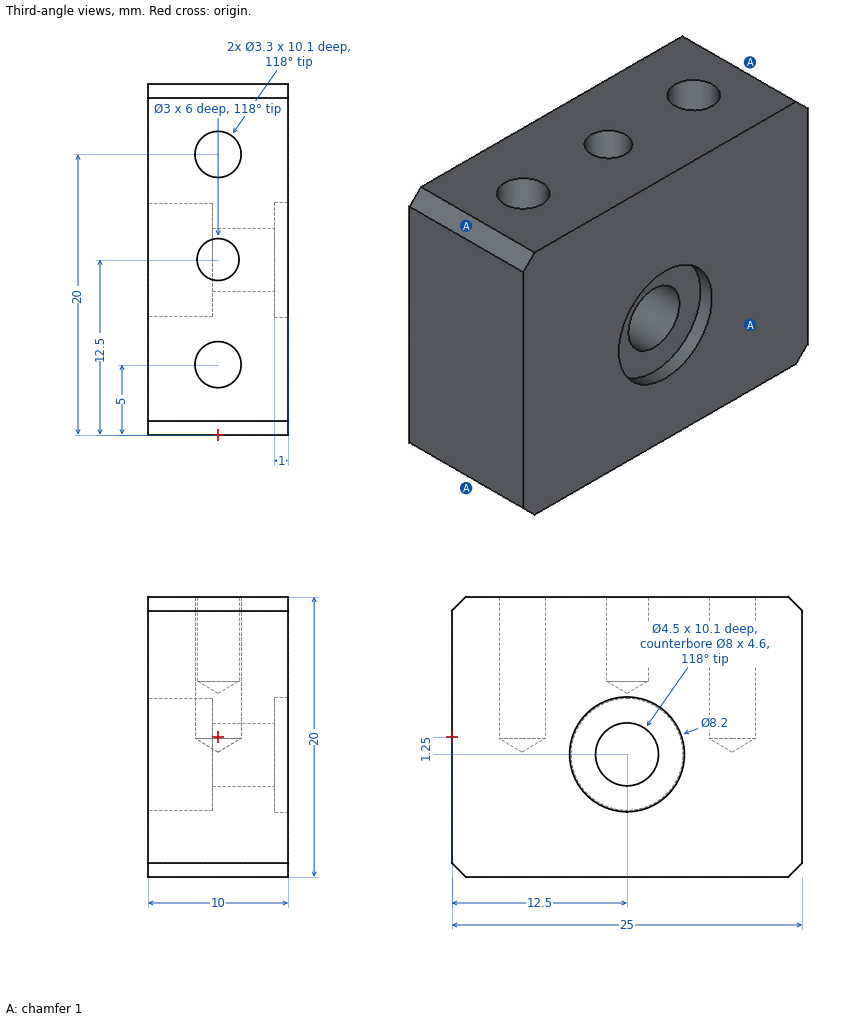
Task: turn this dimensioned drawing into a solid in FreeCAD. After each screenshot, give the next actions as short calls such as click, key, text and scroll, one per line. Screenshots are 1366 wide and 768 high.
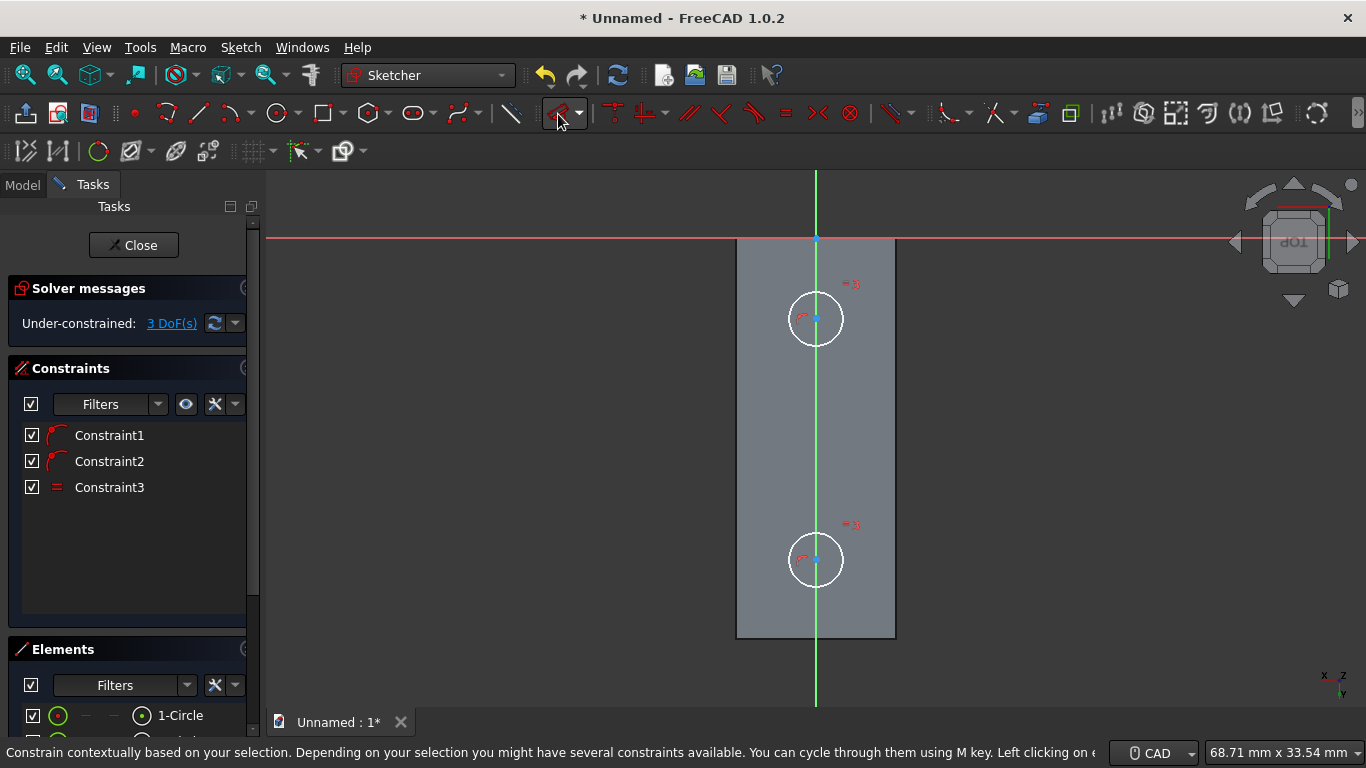
click(835, 541)
click(858, 518)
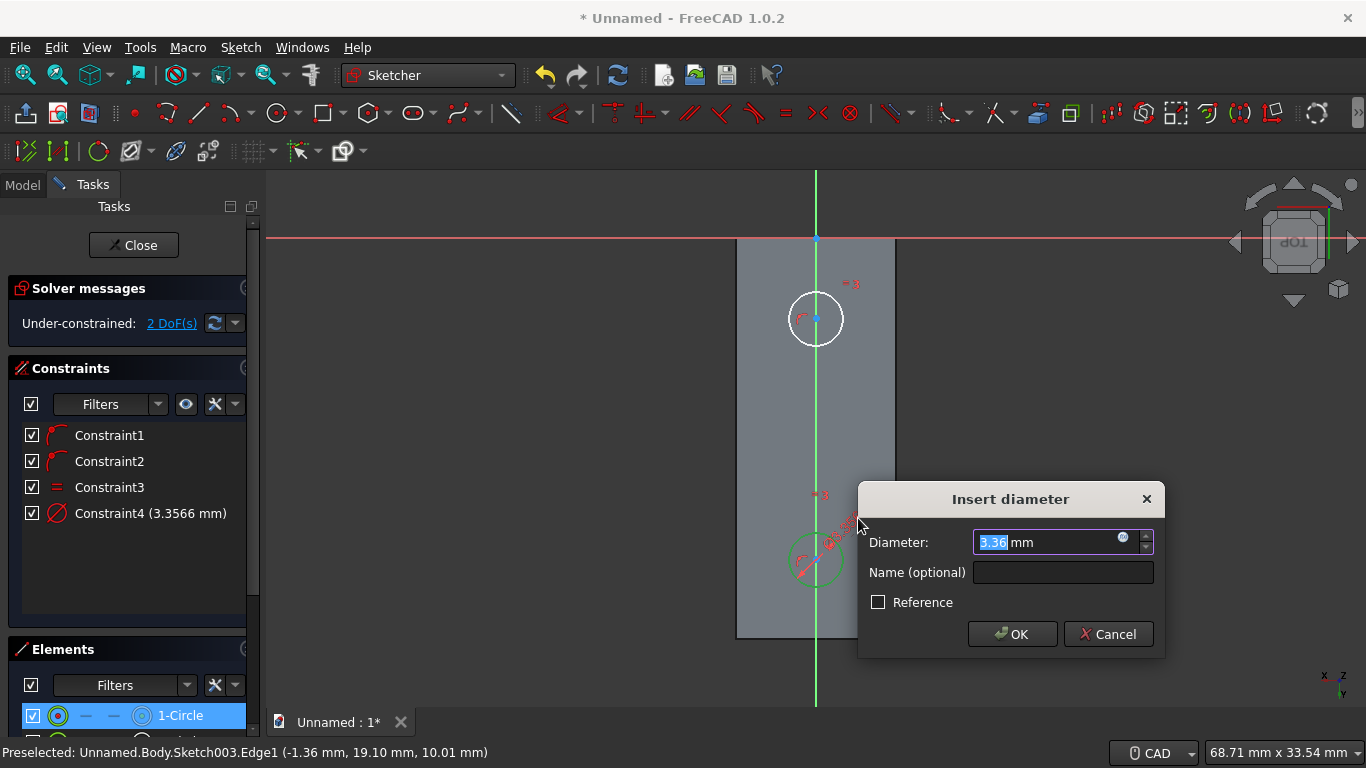
text(3.3)
key(Return)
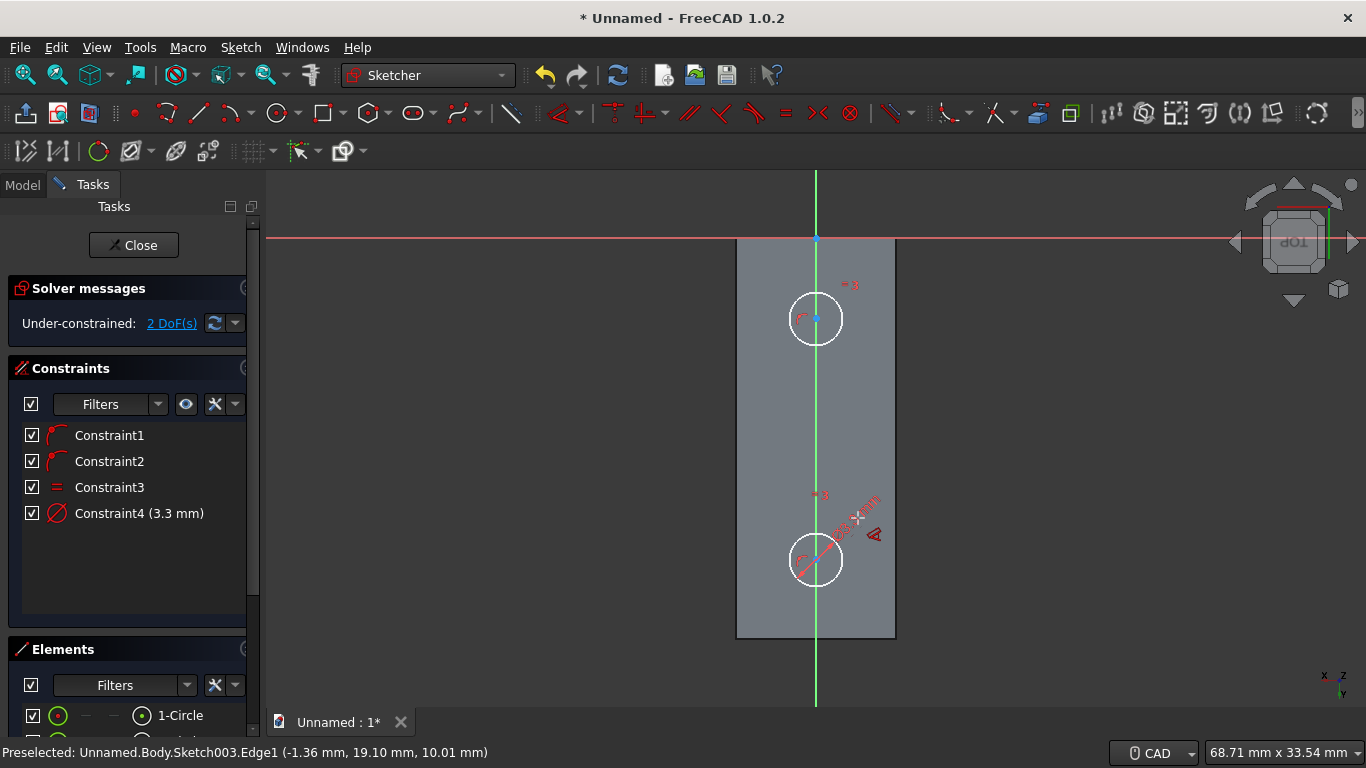
click(816, 319)
click(850, 279)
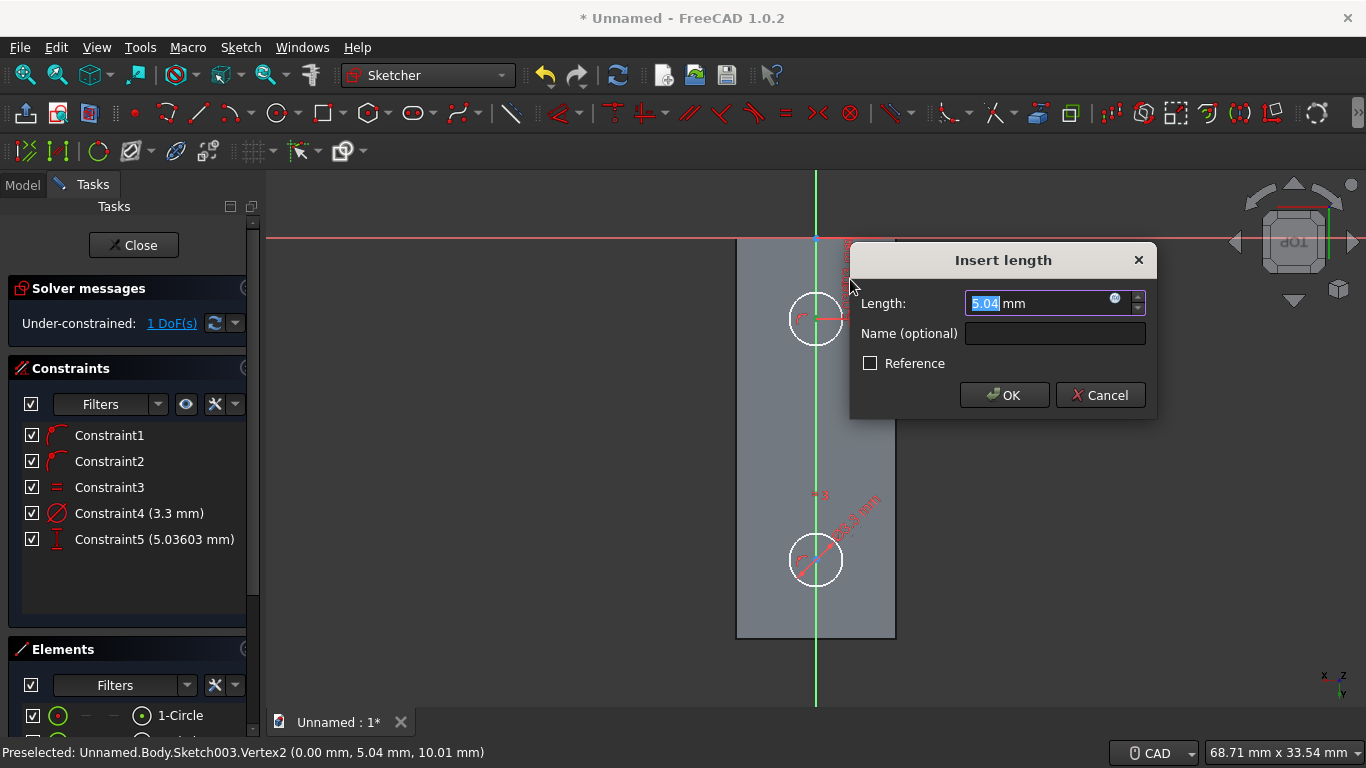
text(5)
key(Return)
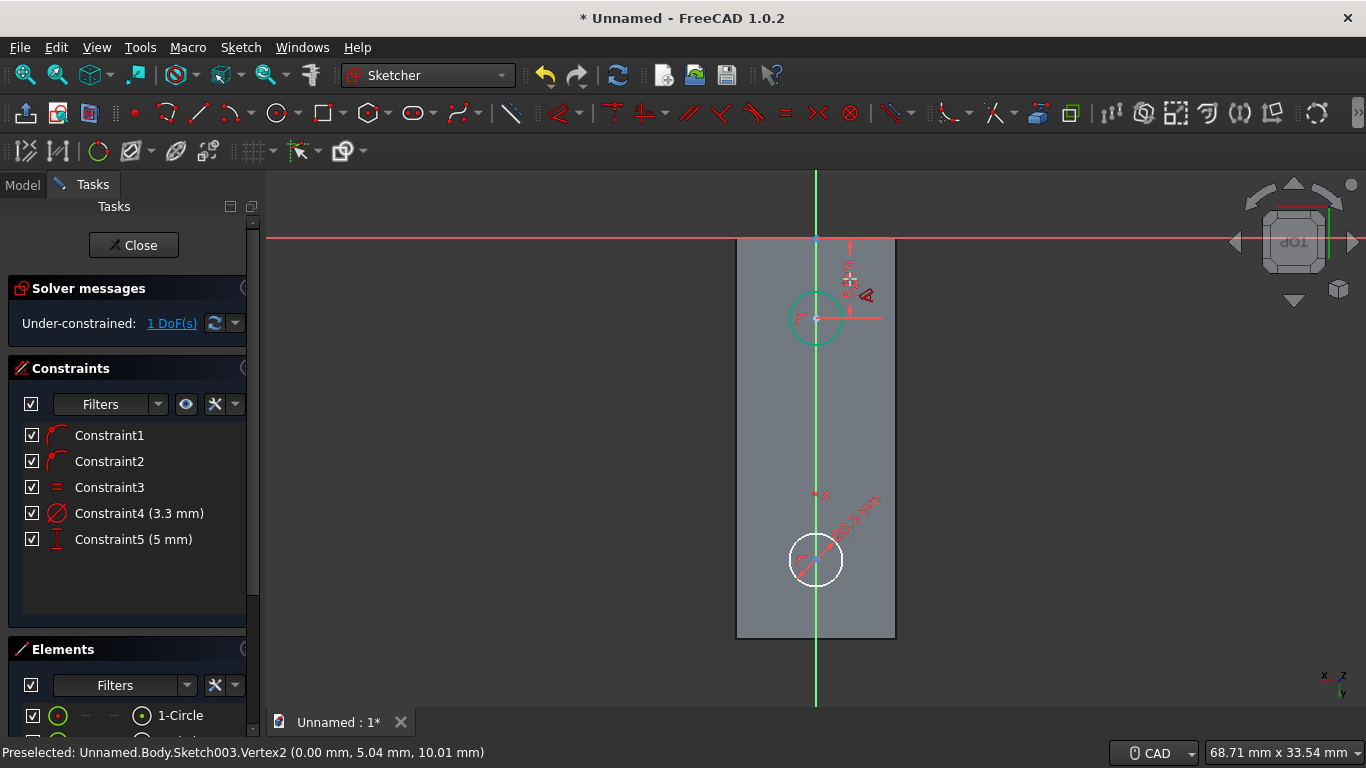
click(816, 560)
click(850, 399)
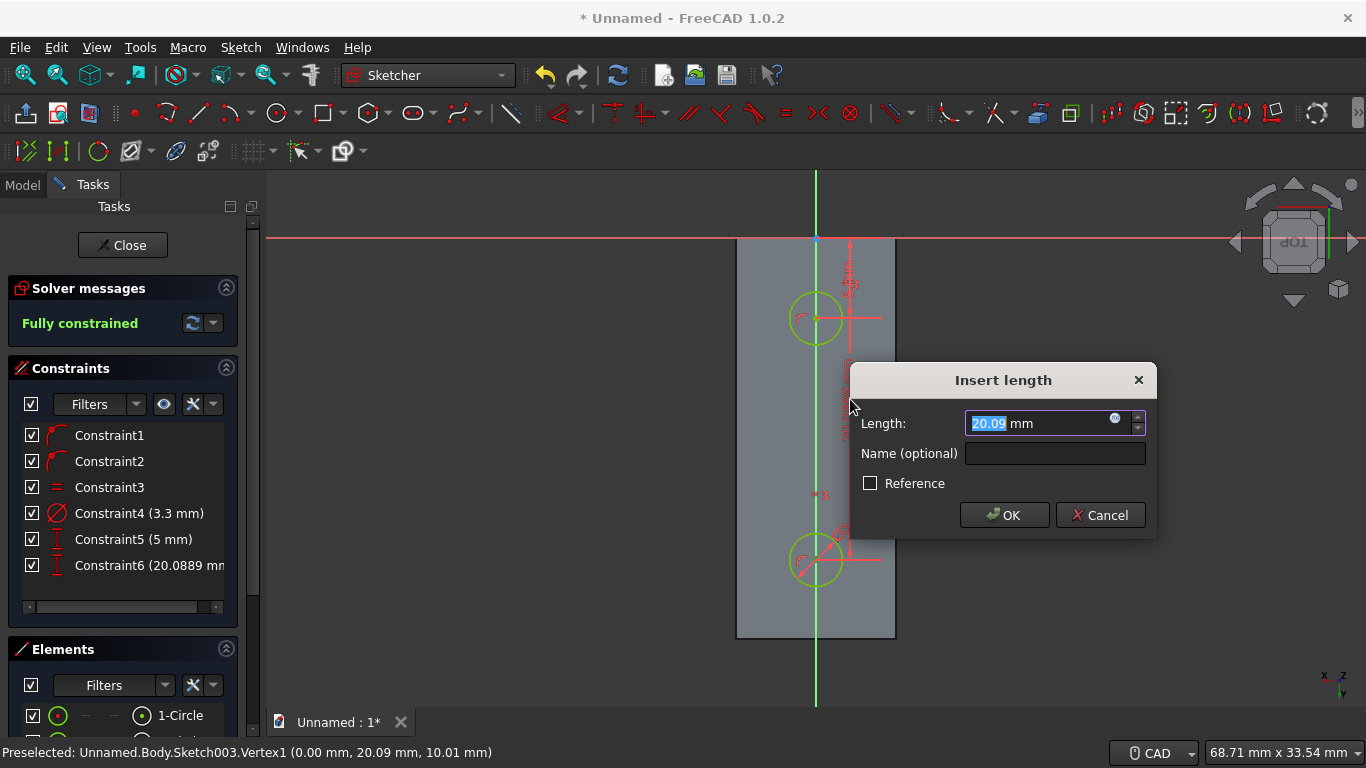
text(20)
key(Return)
key(Escape)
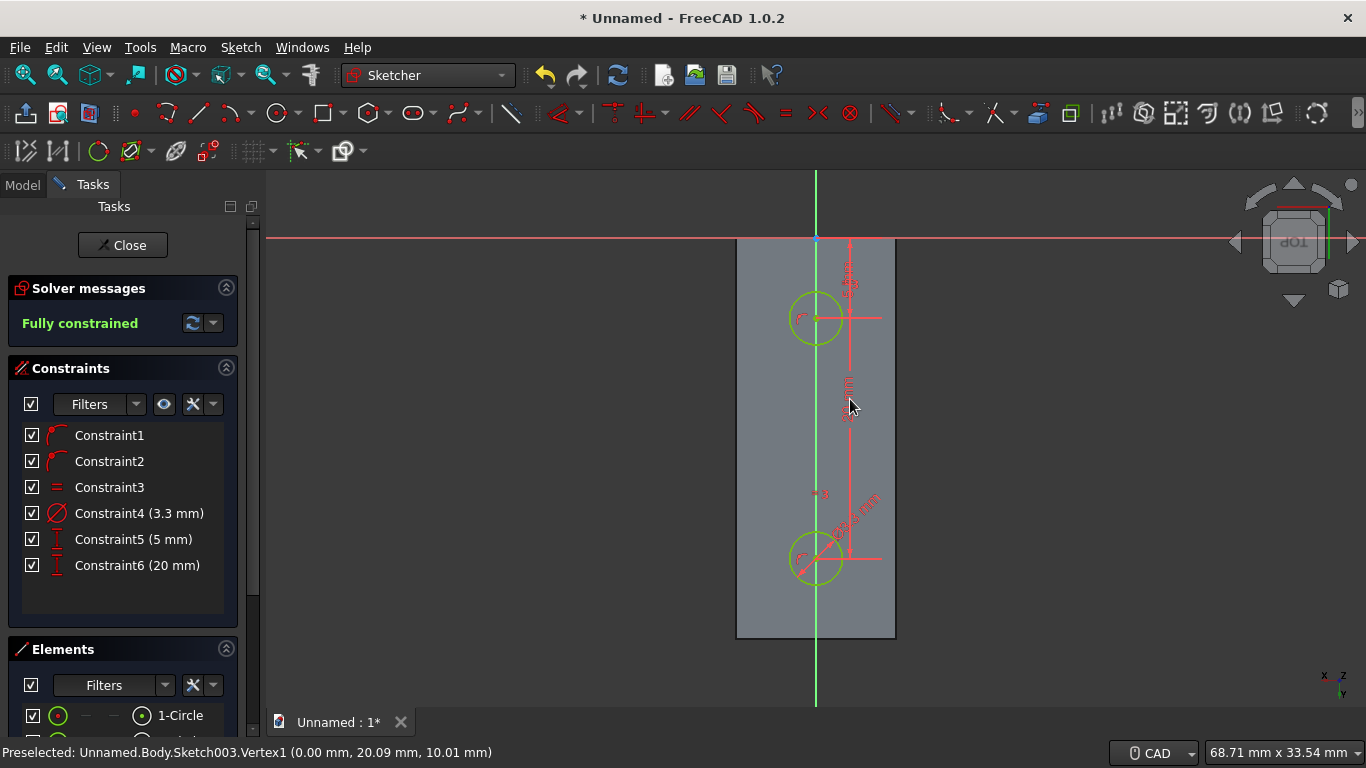
click(123, 245)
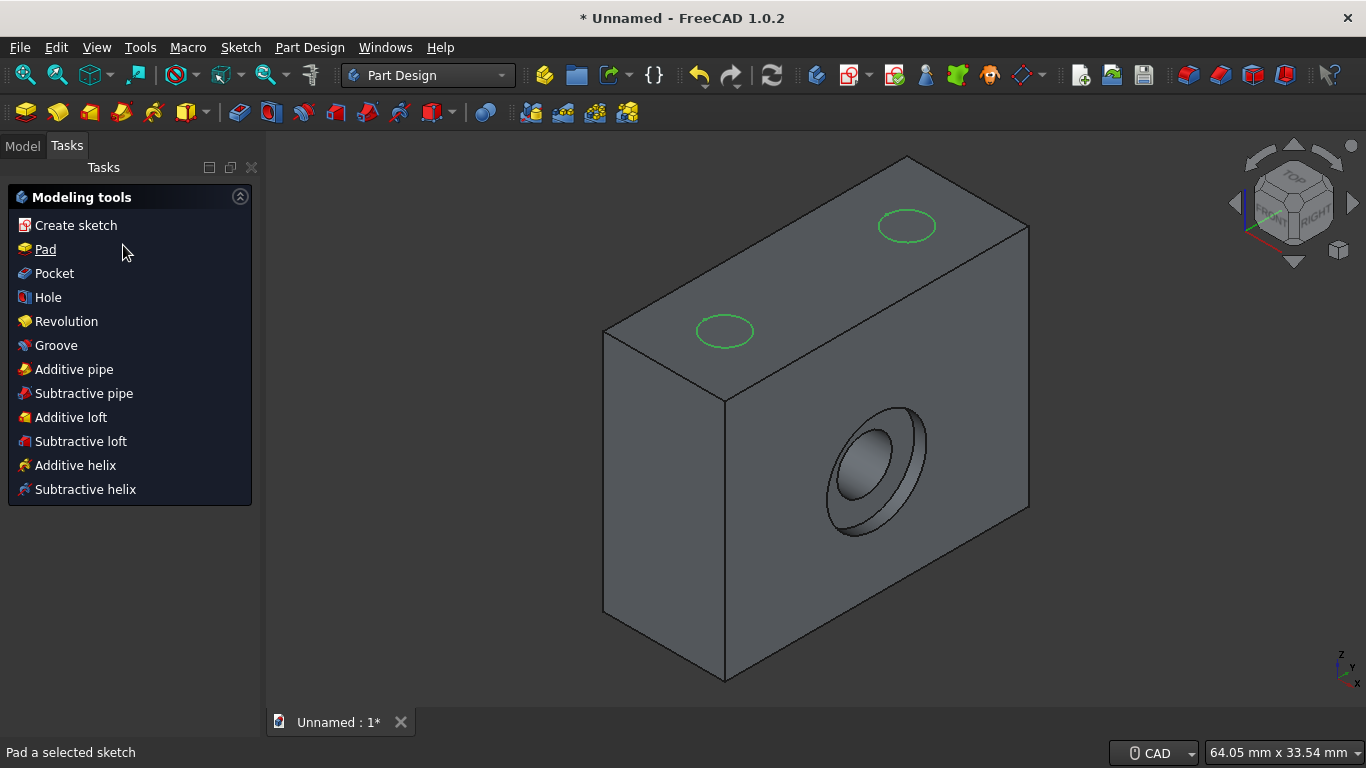
click(272, 112)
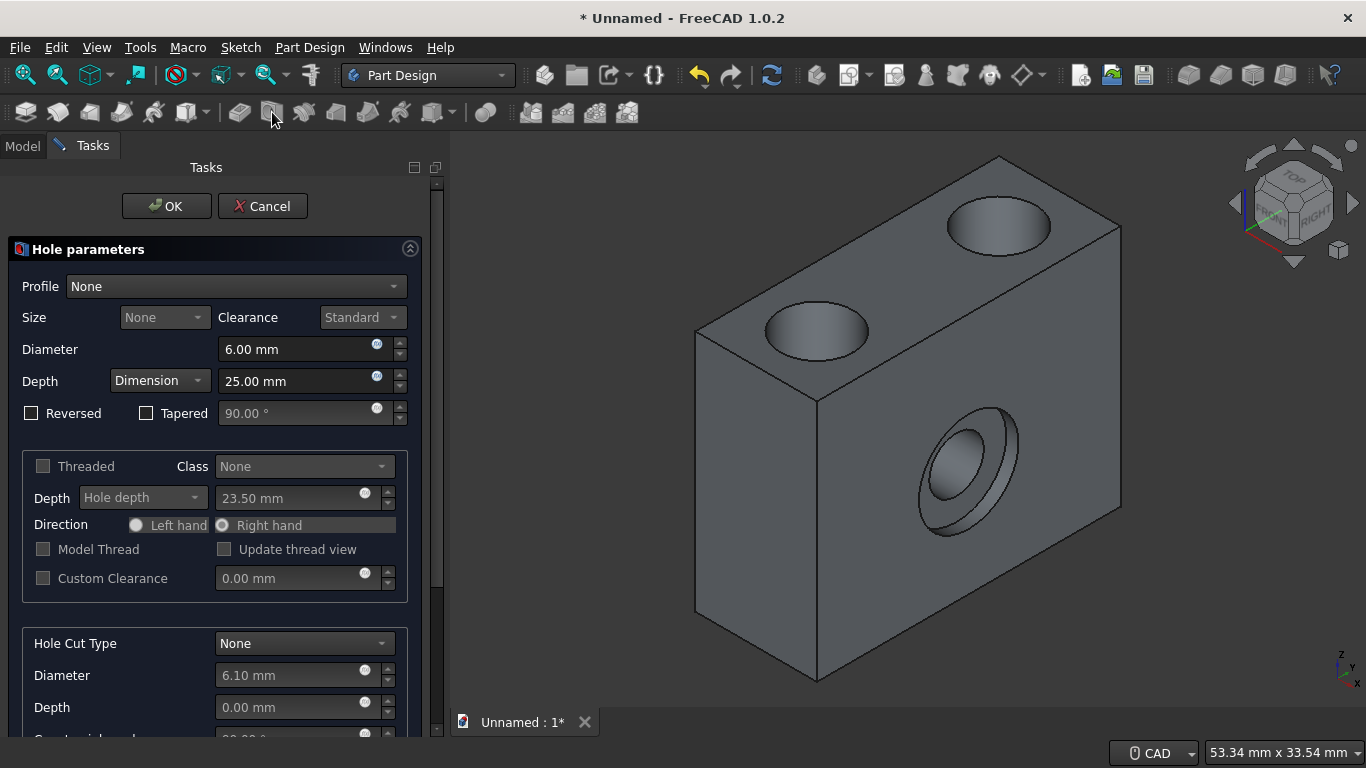
triple_click(305, 349)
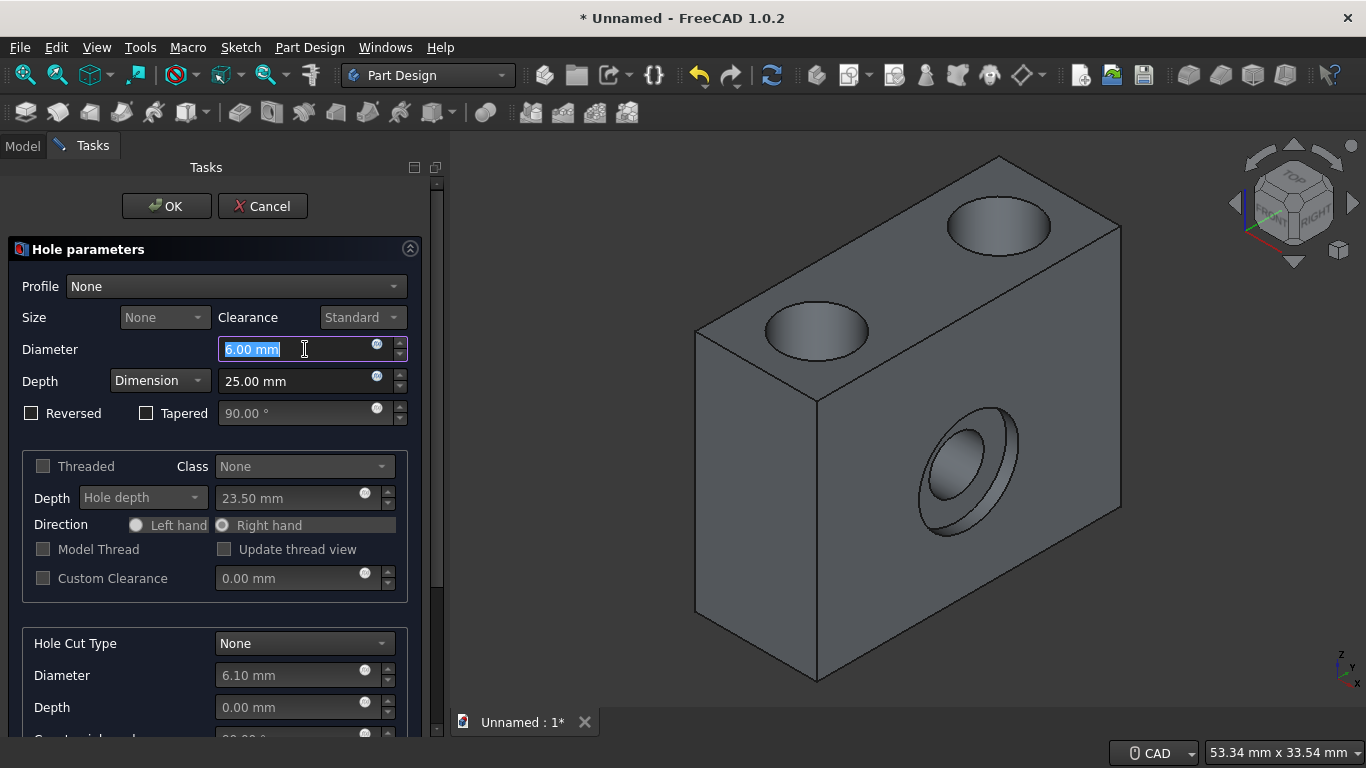
text(3.3)
key(Tab)